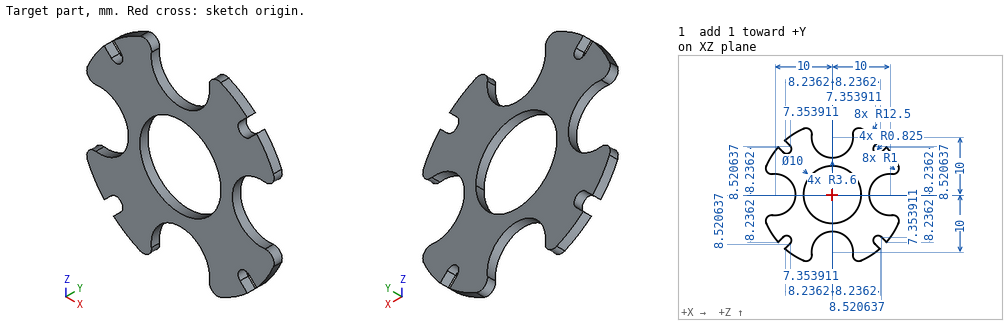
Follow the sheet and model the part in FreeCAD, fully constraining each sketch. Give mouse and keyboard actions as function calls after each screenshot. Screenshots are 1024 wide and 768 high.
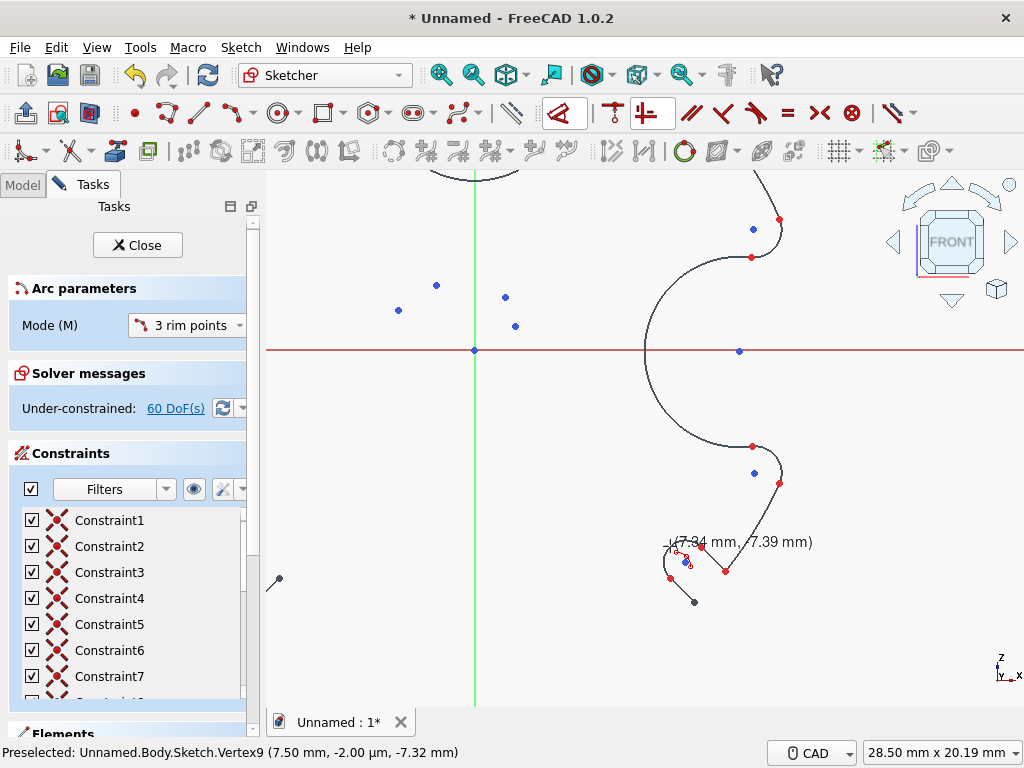
click(695, 602)
click(607, 656)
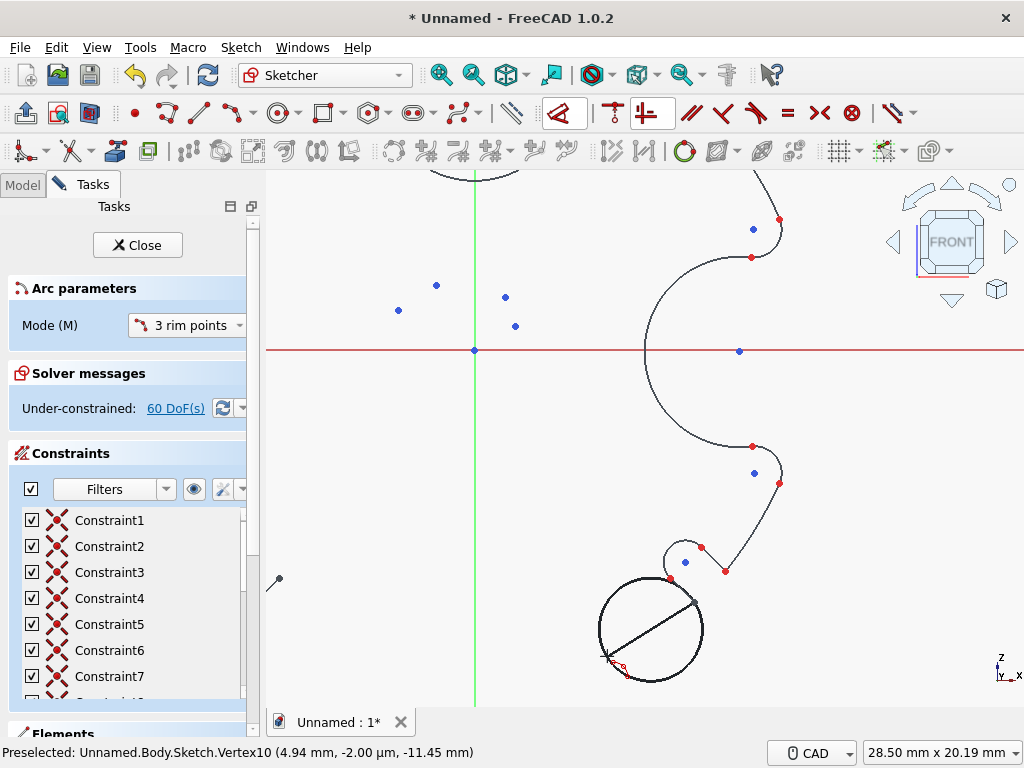
scroll(652, 631, up, 7)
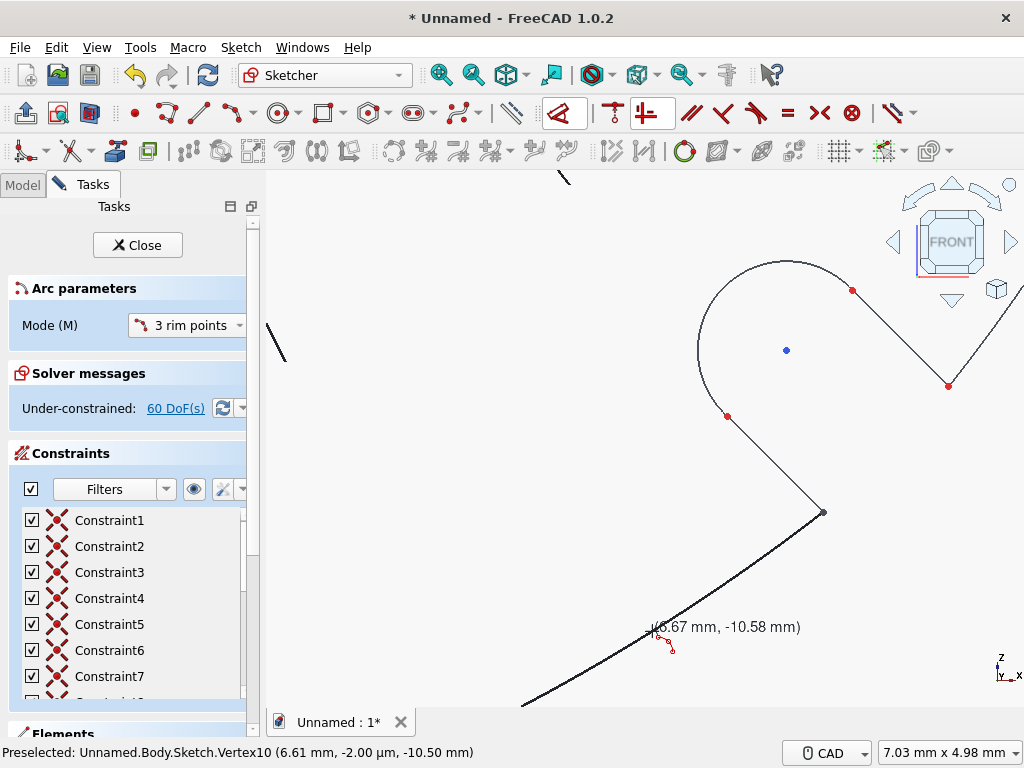
click(652, 630)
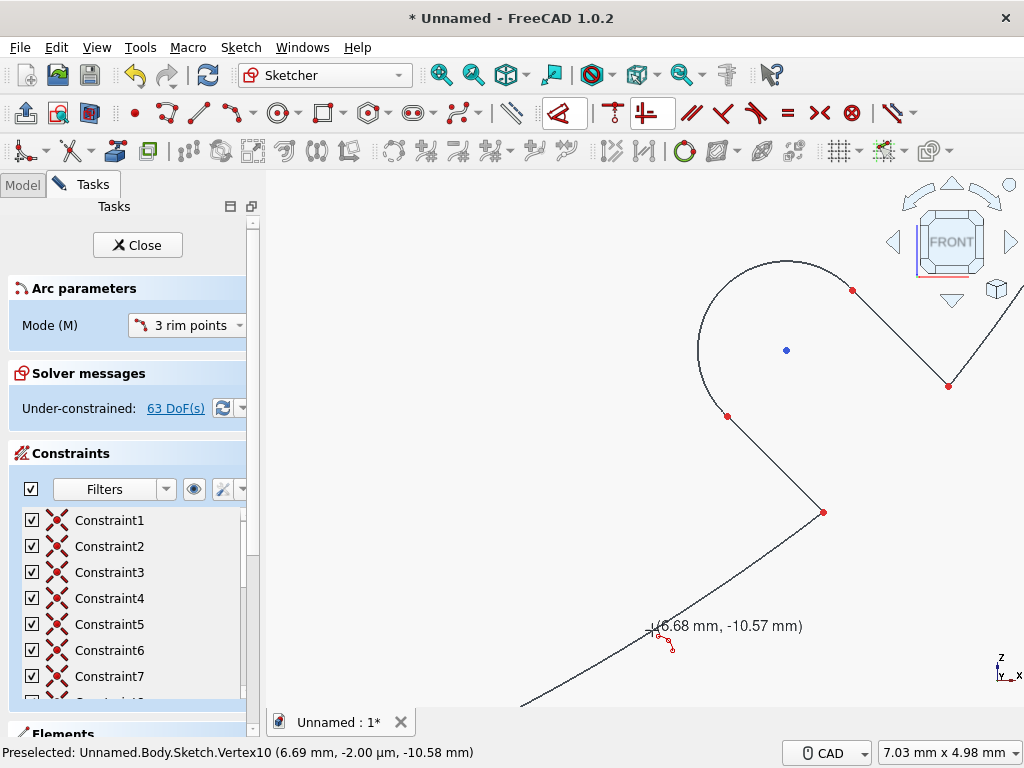
scroll(677, 587, down, 10)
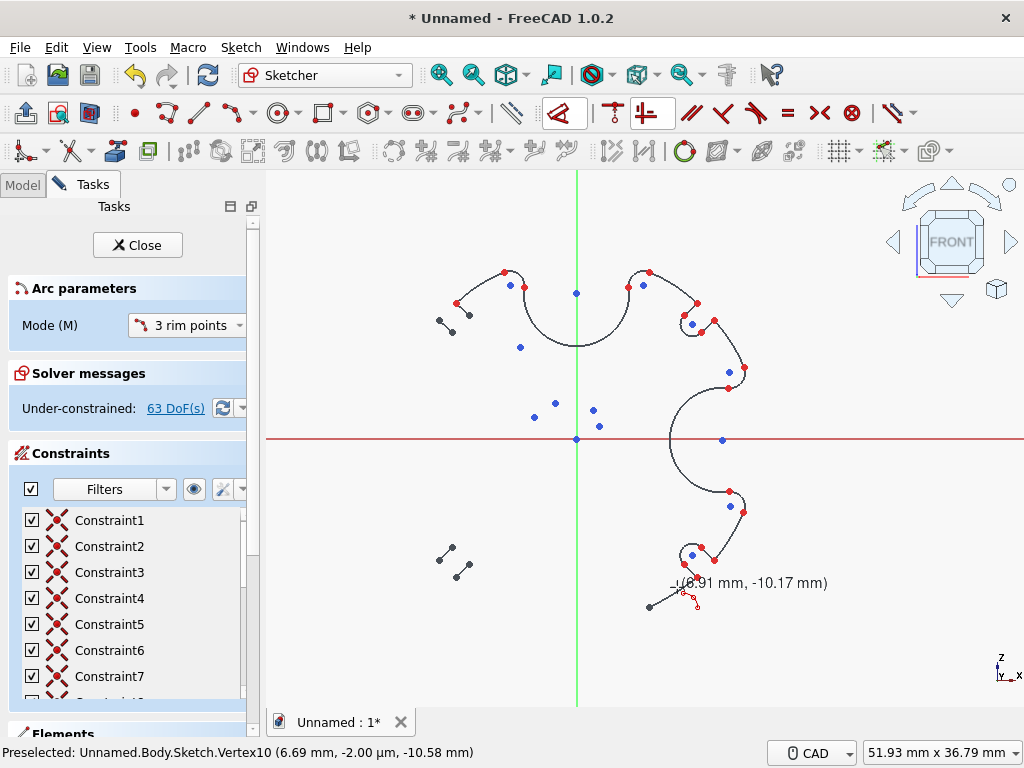
click(649, 608)
click(629, 592)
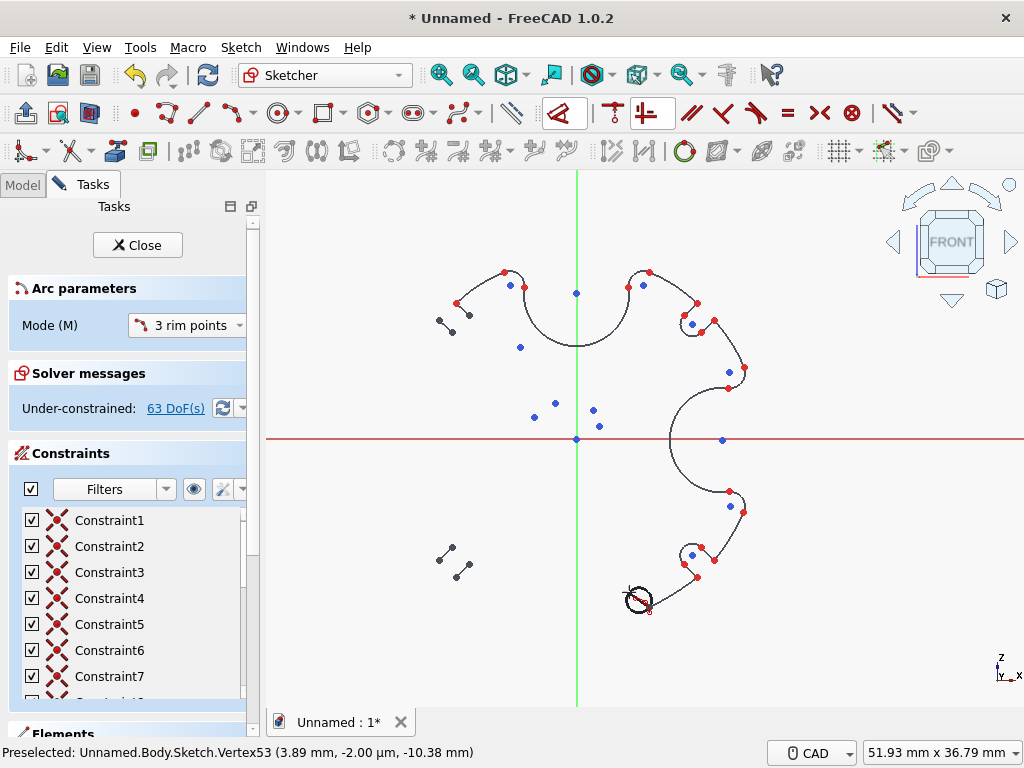
scroll(634, 605, up, 4)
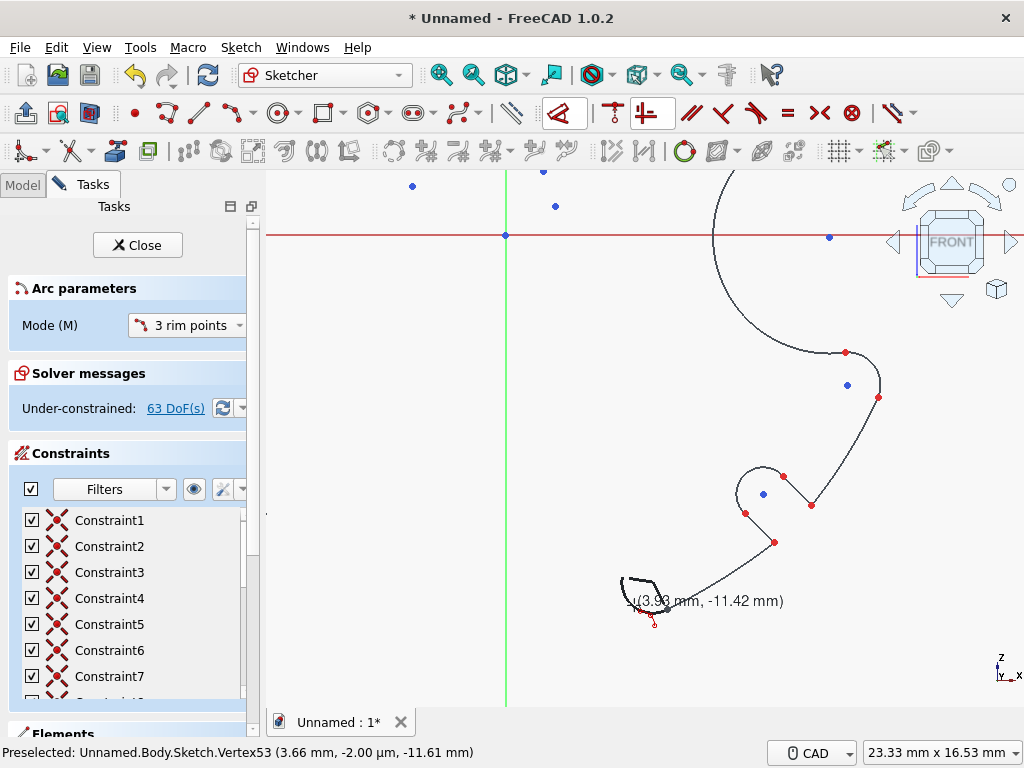
click(634, 604)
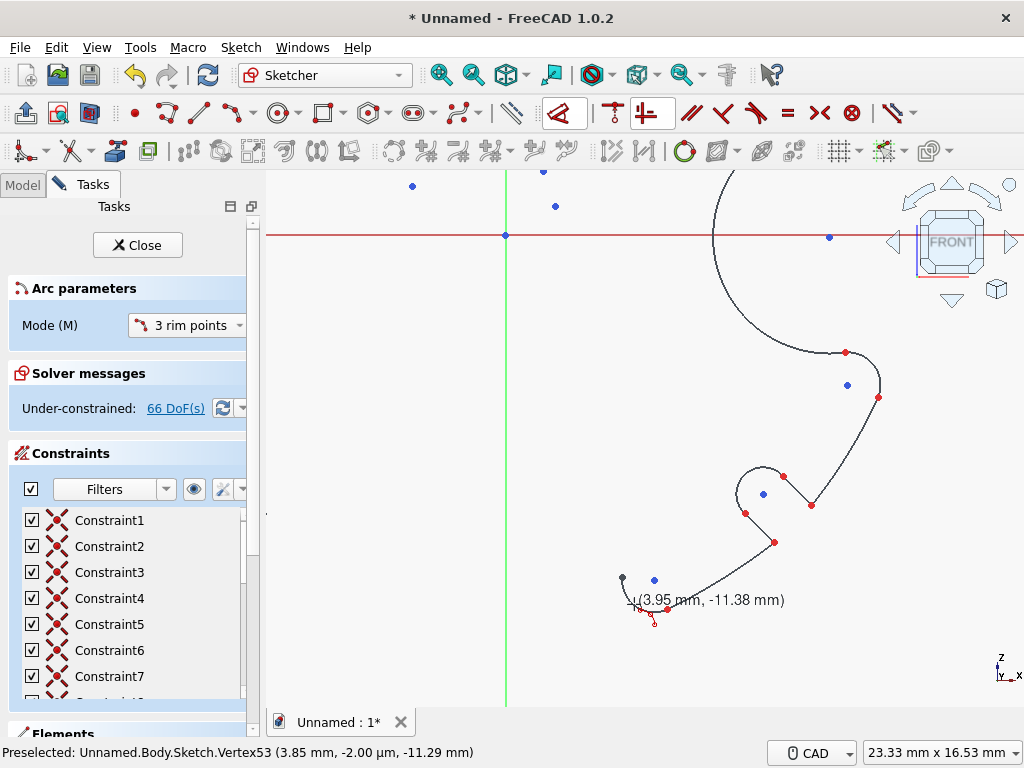
click(622, 577)
click(389, 574)
click(544, 450)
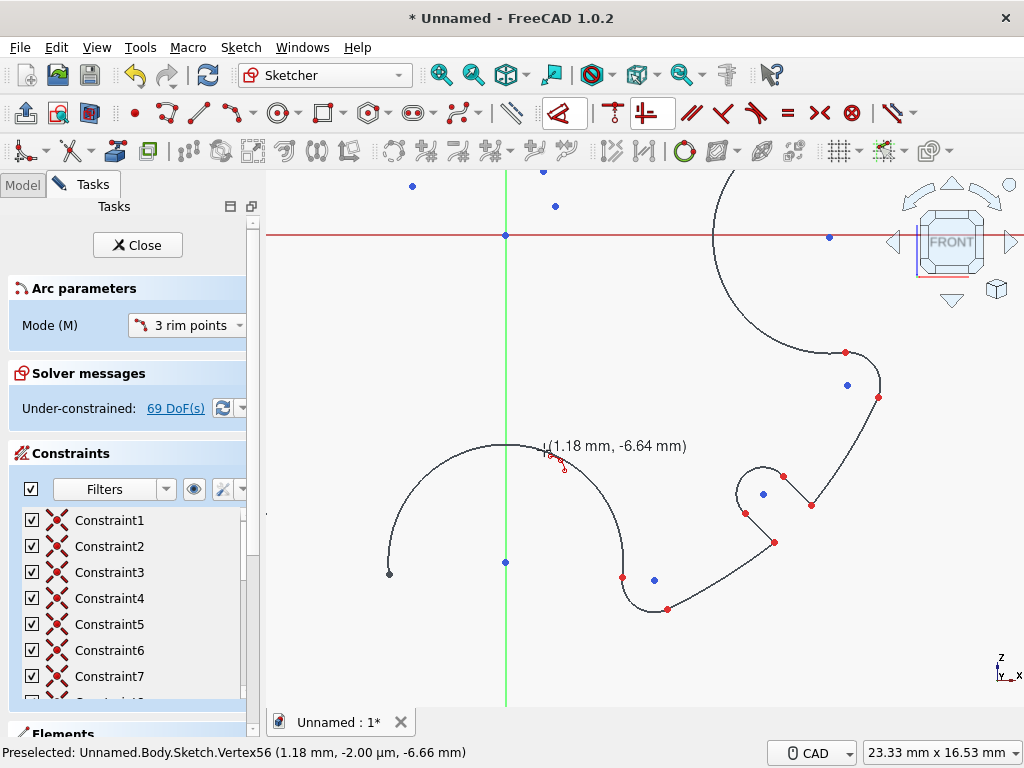
click(389, 575)
click(344, 608)
click(377, 604)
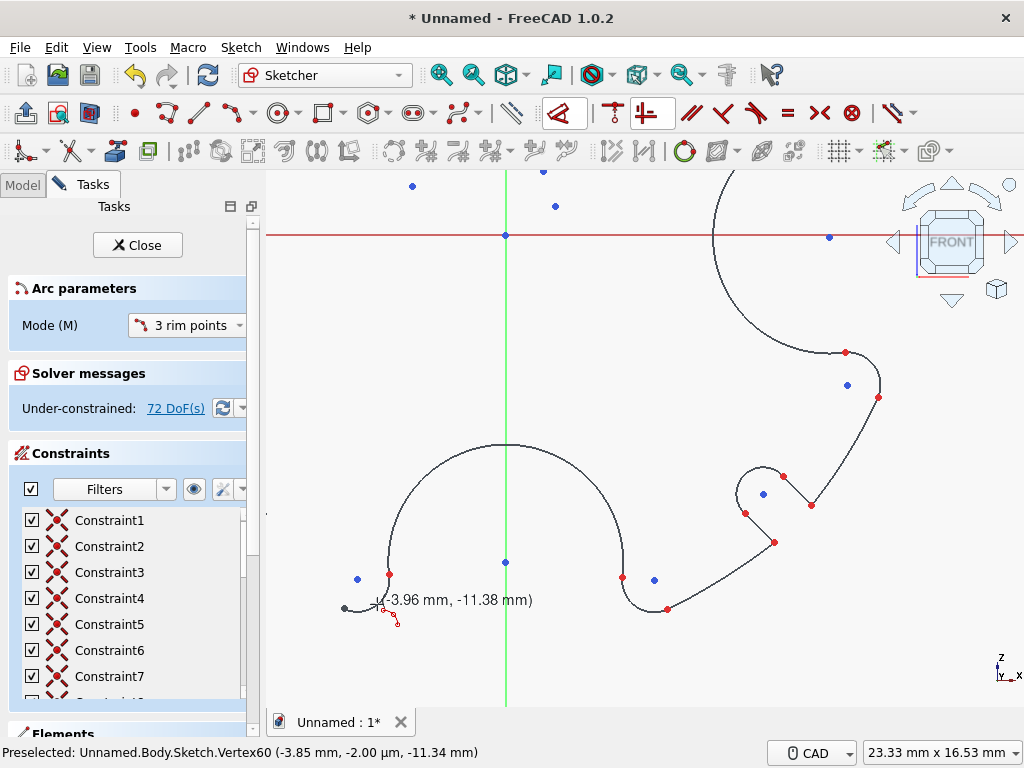
click(344, 609)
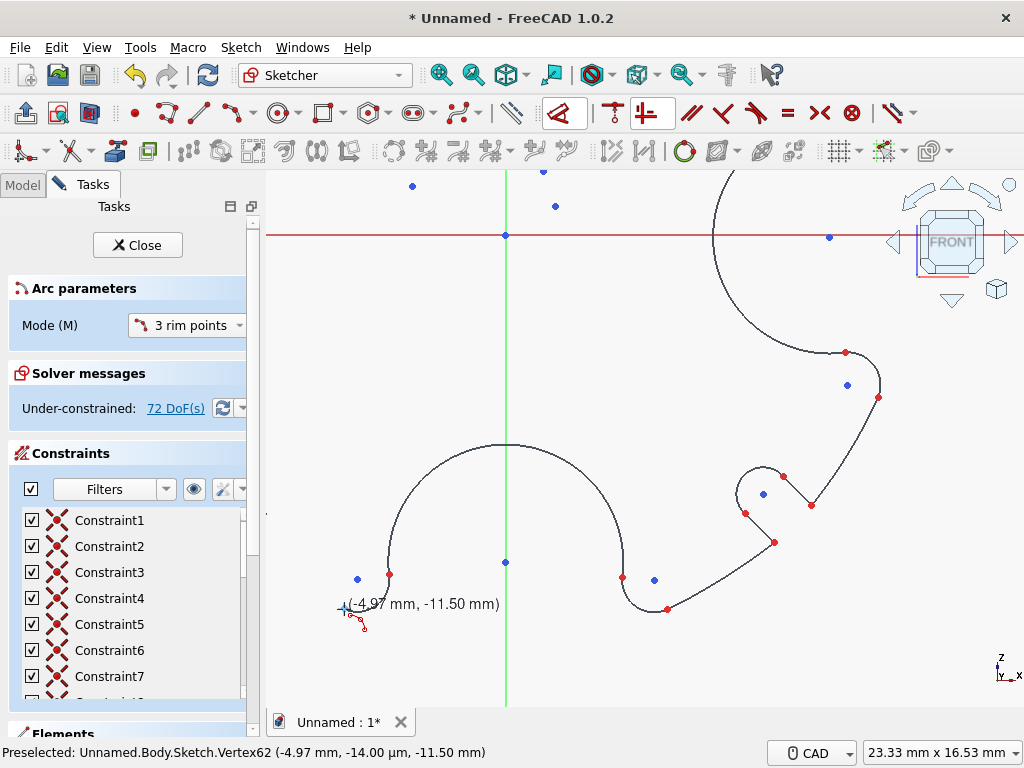
scroll(634, 604, down, 4)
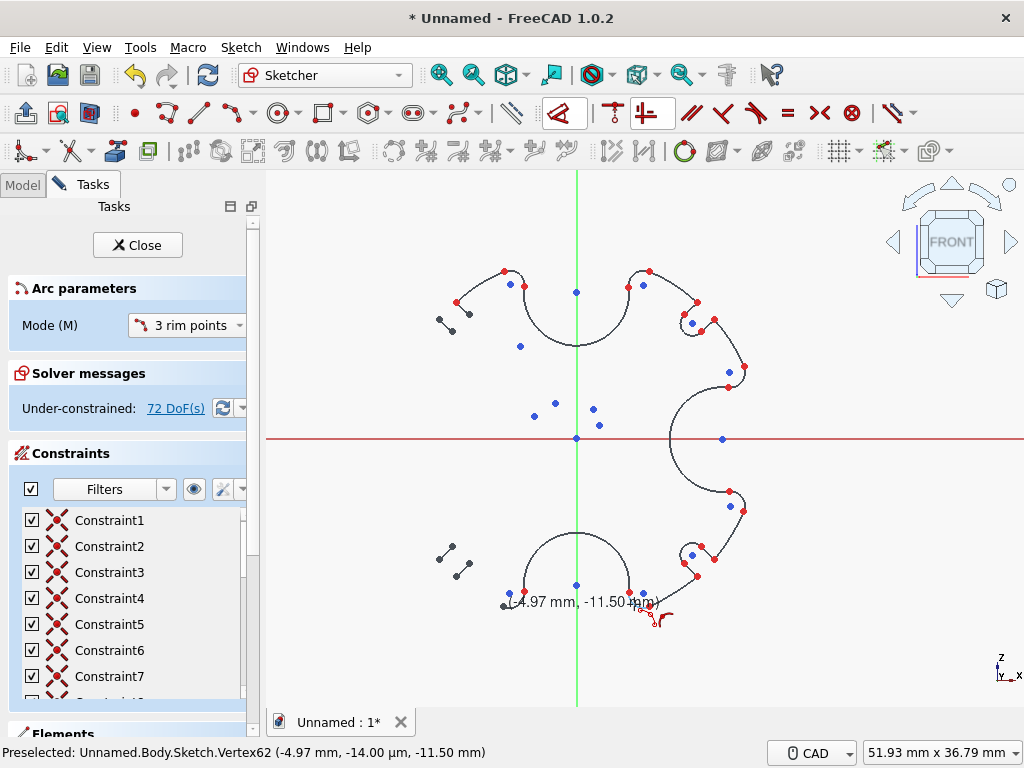
scroll(456, 576, up, 3)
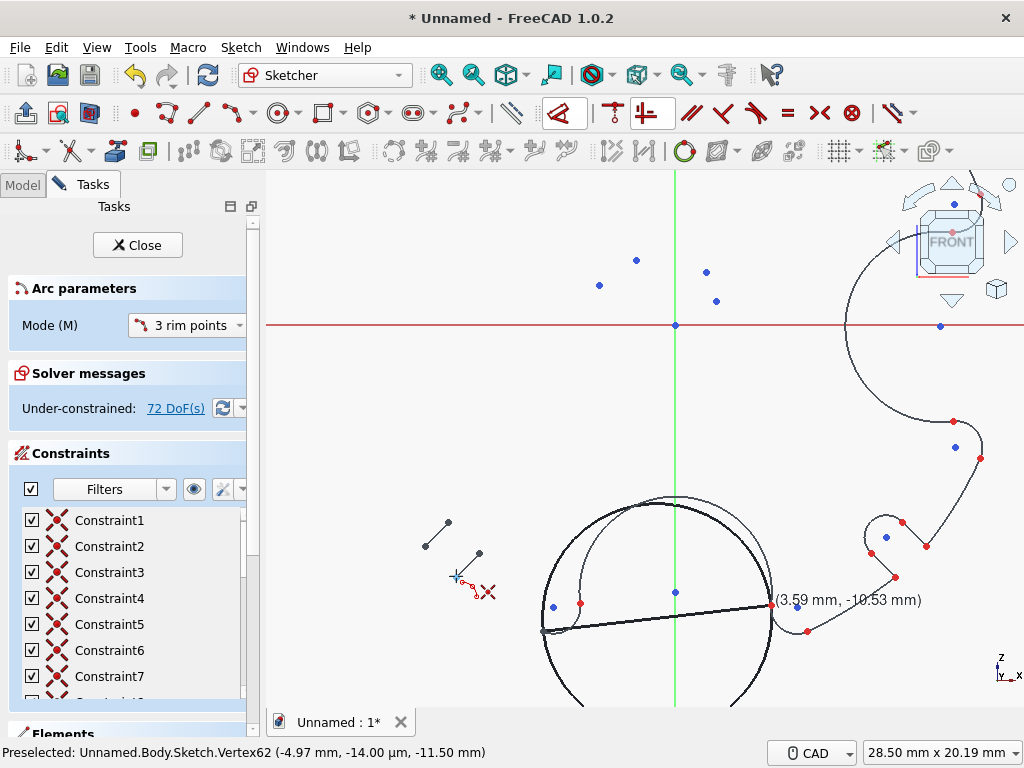
click(456, 577)